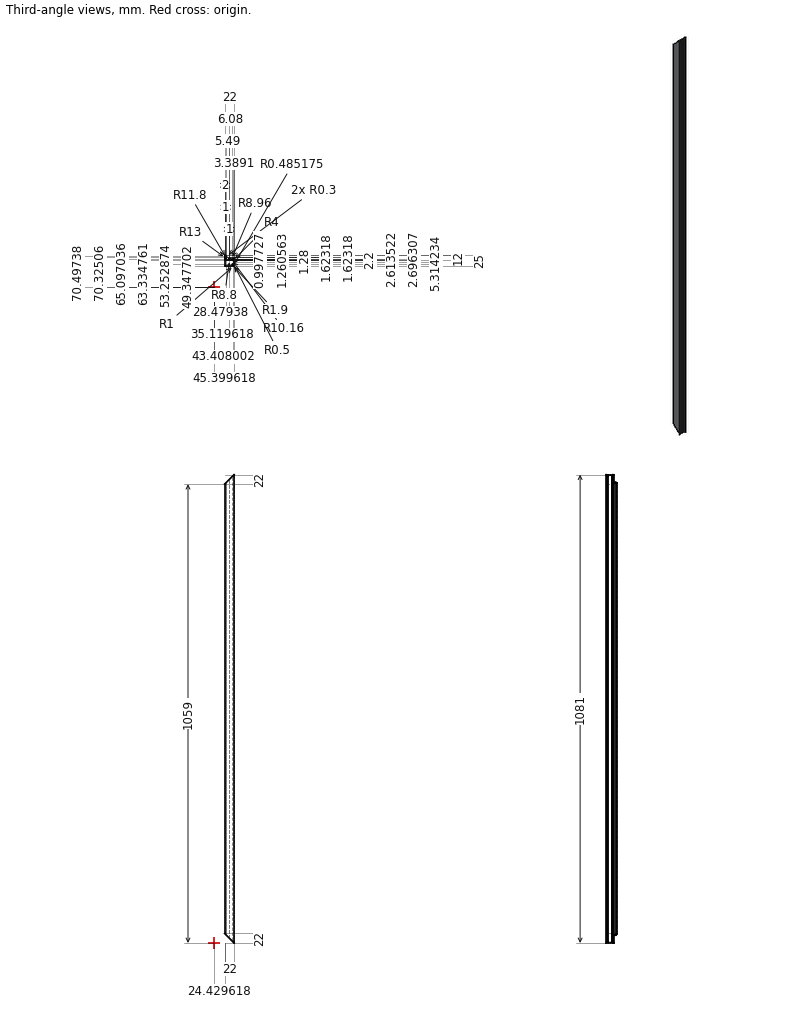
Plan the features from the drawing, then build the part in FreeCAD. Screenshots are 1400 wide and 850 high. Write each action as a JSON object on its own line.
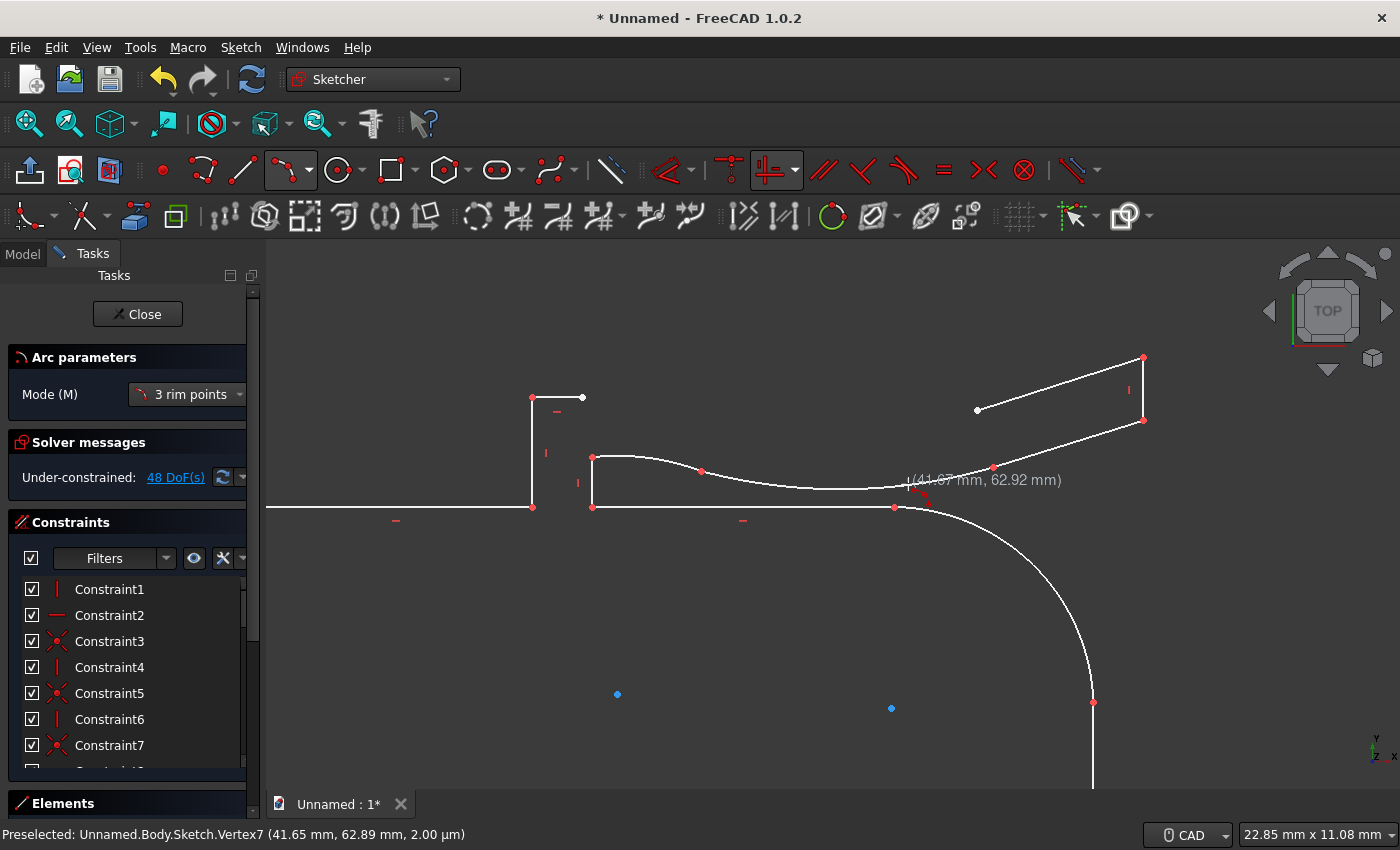
{"action": "left_click", "coordinate": [977, 411]}
{"action": "left_click", "coordinate": [719, 412]}
{"action": "left_click", "coordinate": [848, 429]}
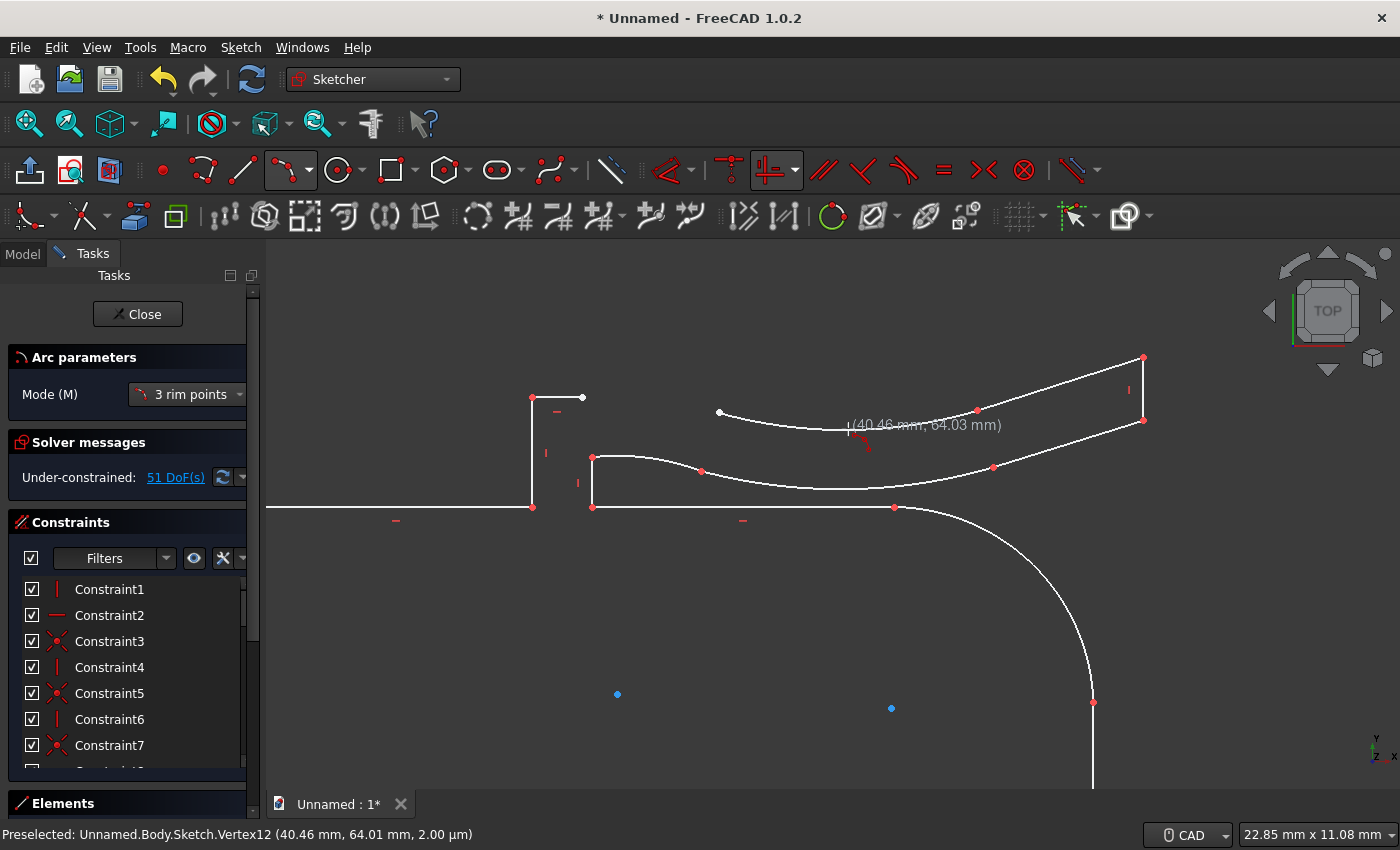
{"action": "left_click", "coordinate": [719, 413]}
{"action": "left_click", "coordinate": [582, 397]}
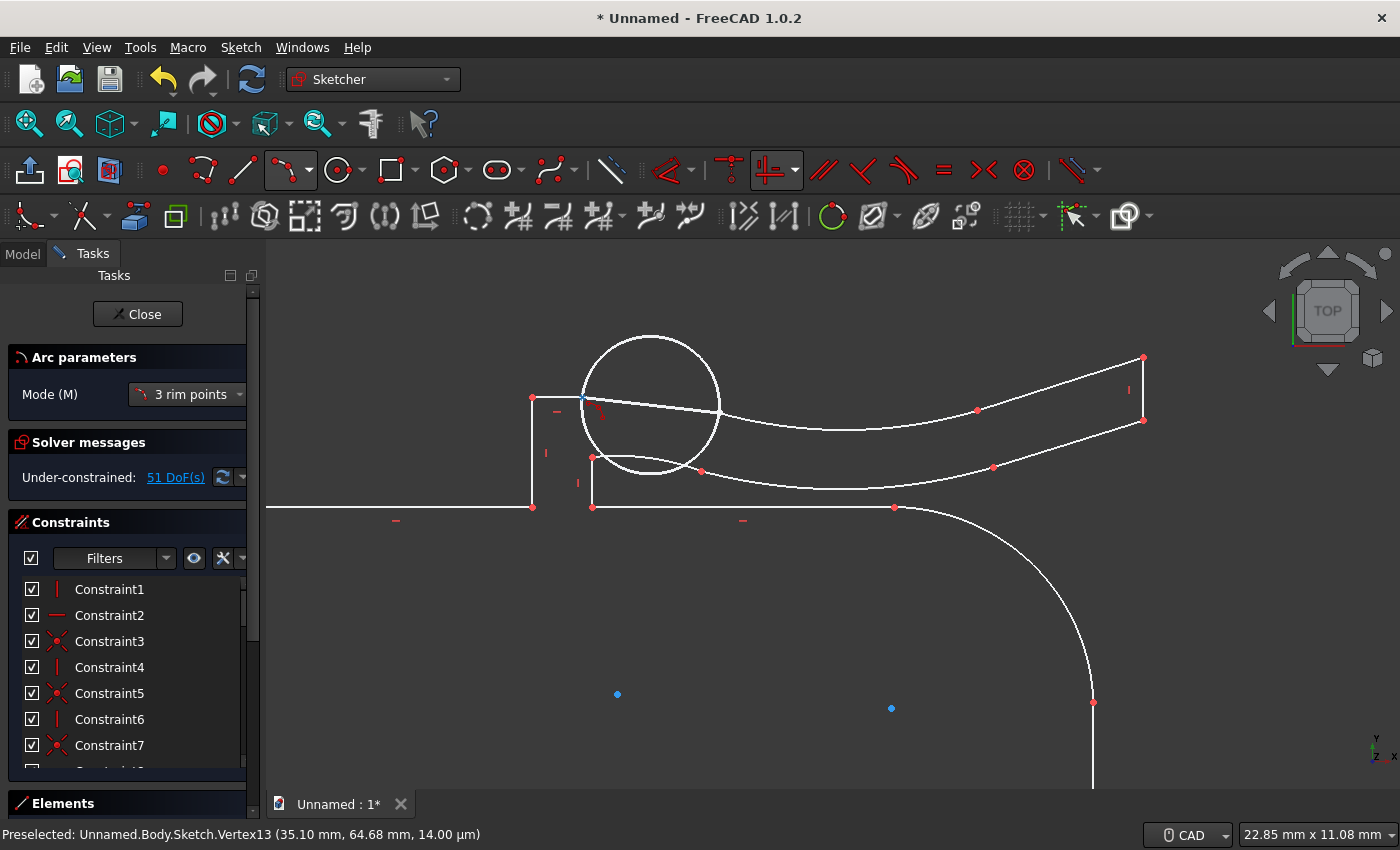
{"action": "scroll", "coordinate": [651, 398], "scroll_direction": "up", "scroll_amount": 7}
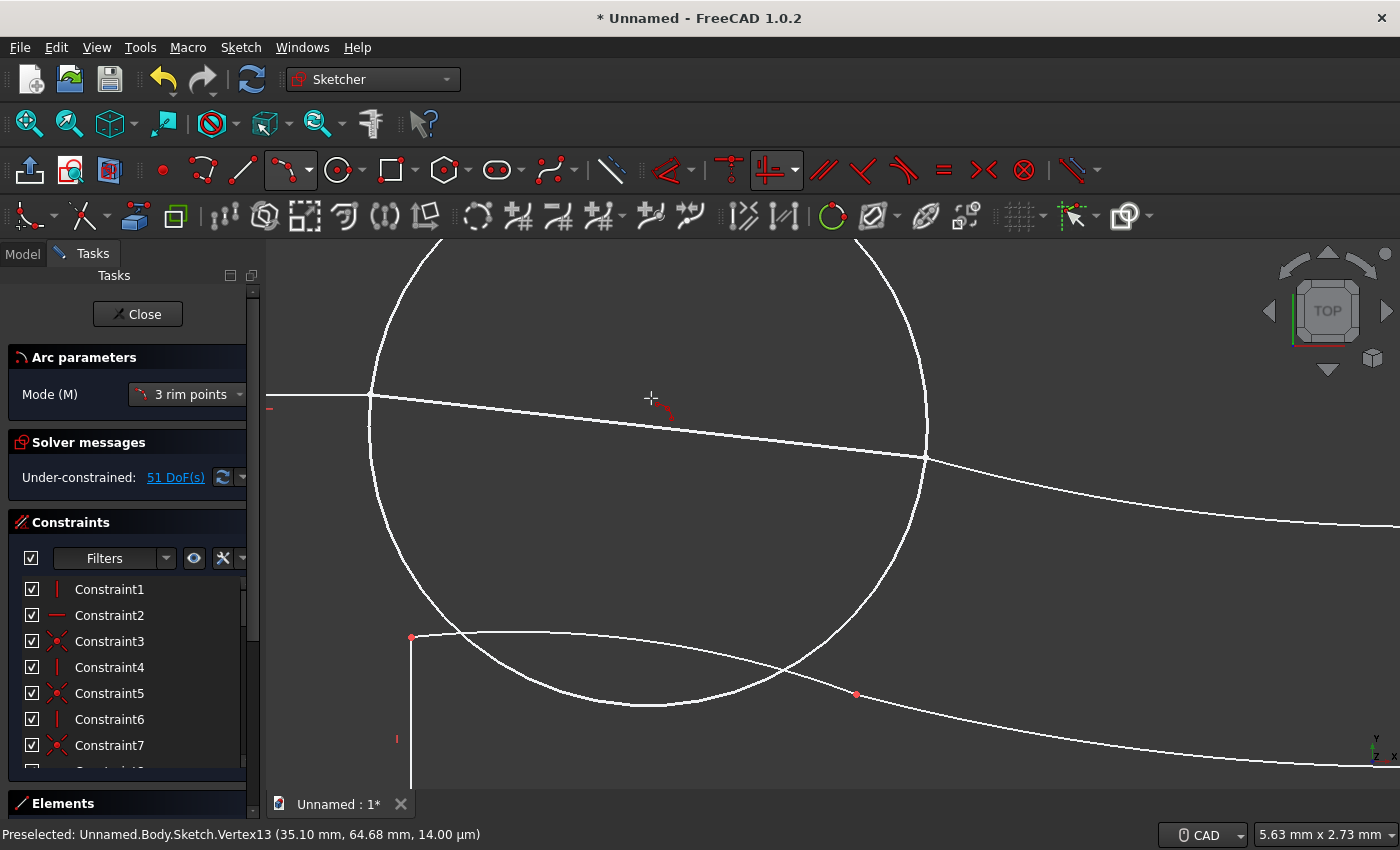
{"action": "left_click", "coordinate": [652, 397]}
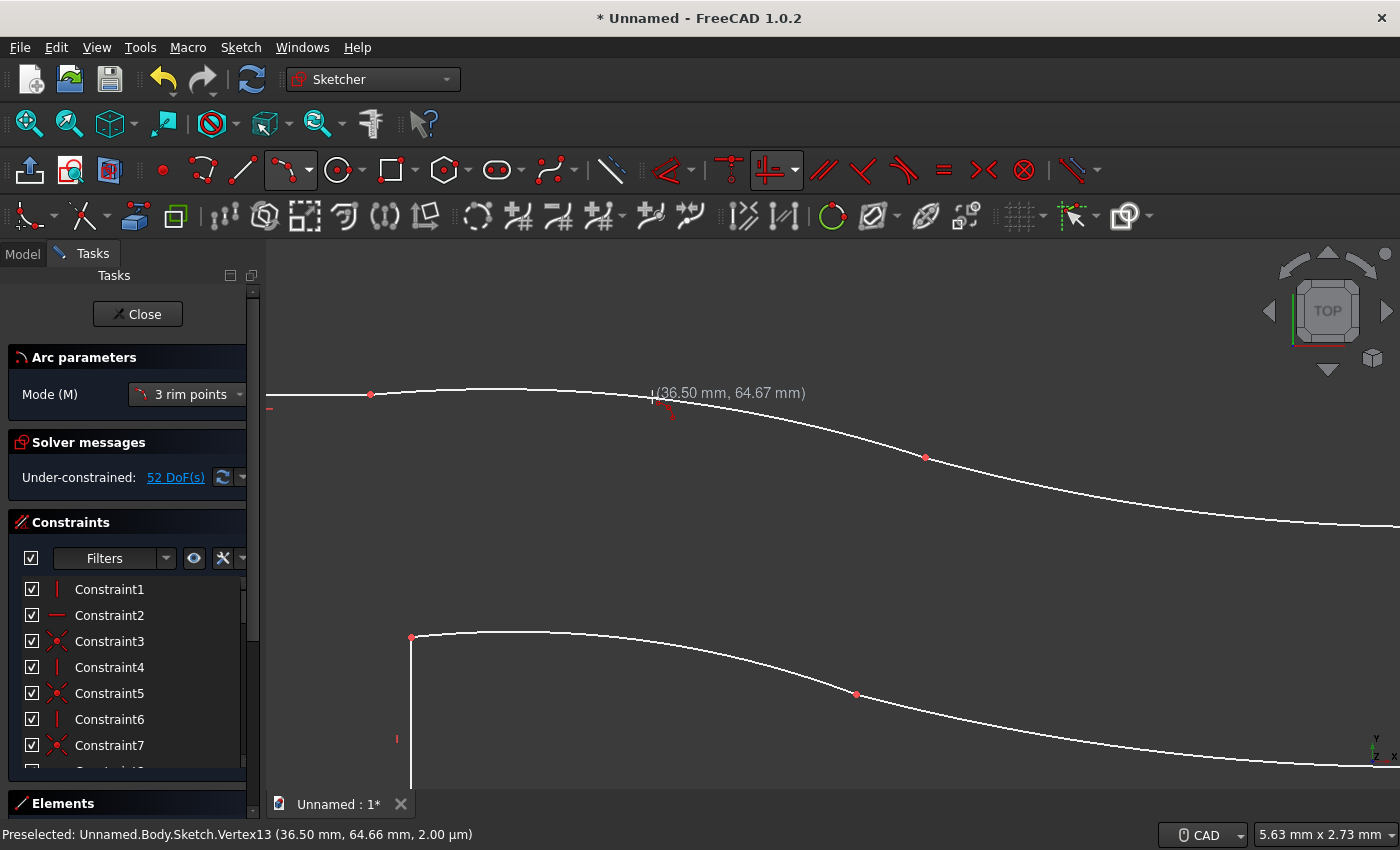
{"action": "scroll", "coordinate": [791, 459], "scroll_direction": "down", "scroll_amount": 13}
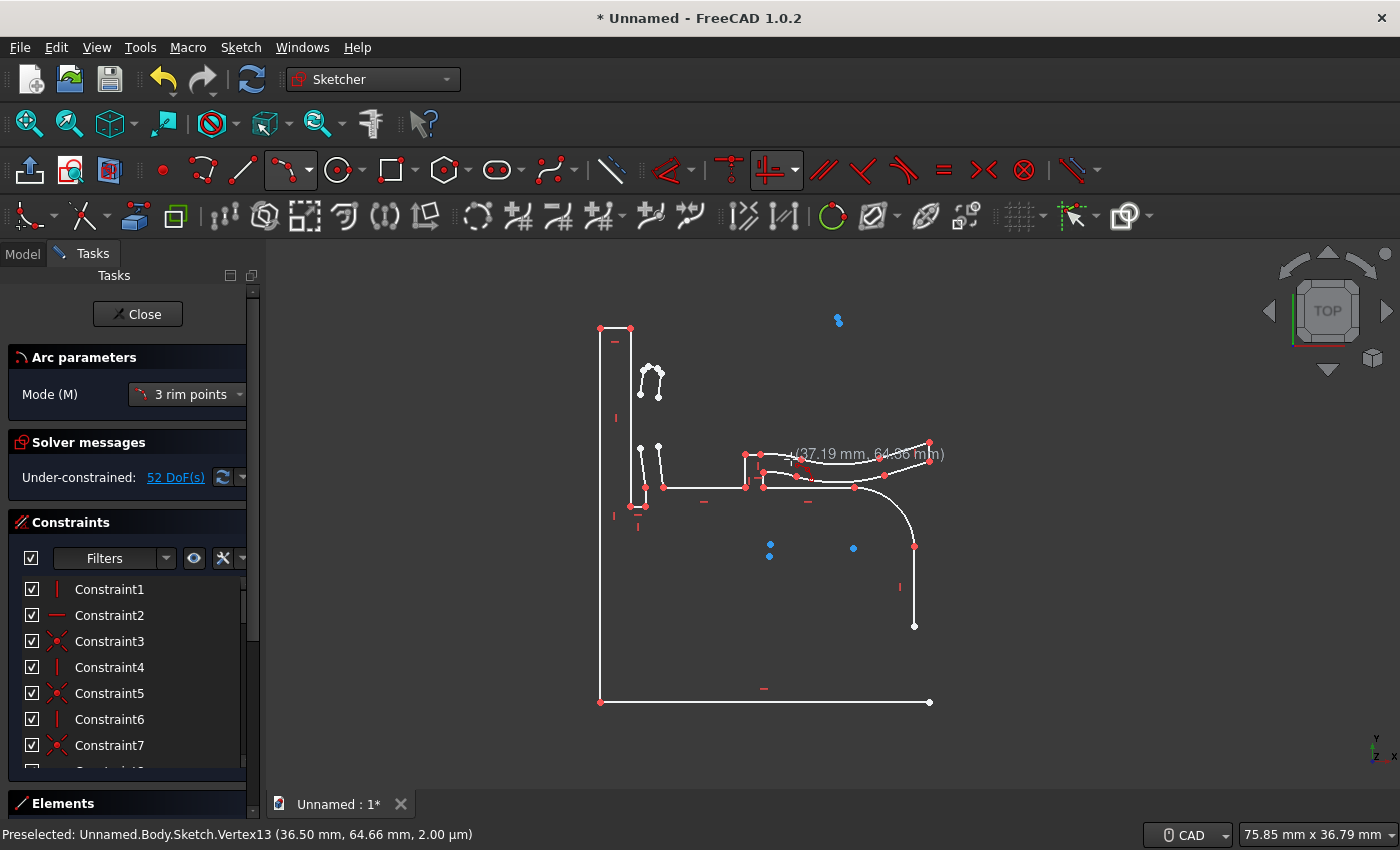
{"action": "left_click", "coordinate": [658, 447]}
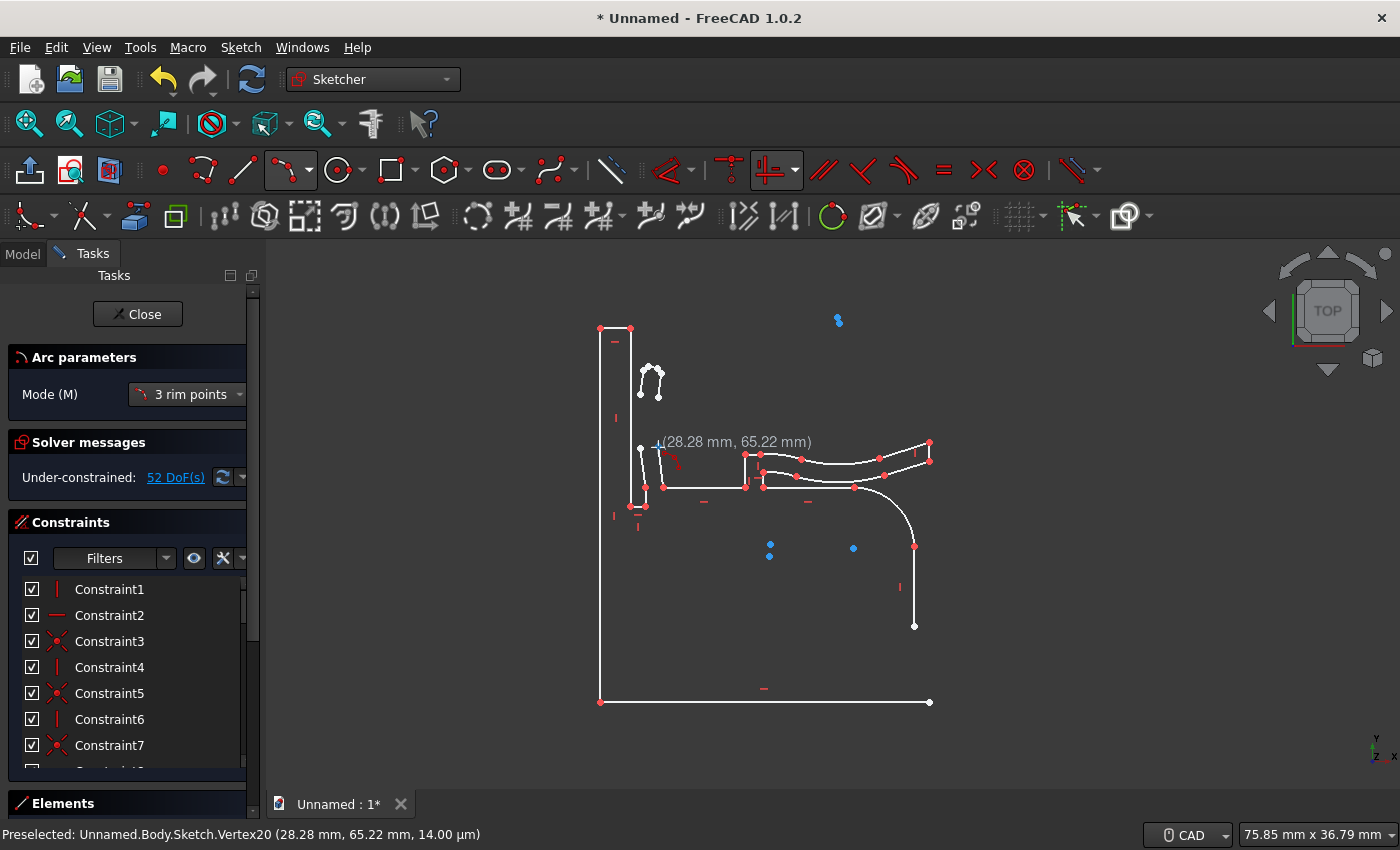
{"action": "scroll", "coordinate": [658, 397], "scroll_direction": "up", "scroll_amount": 2}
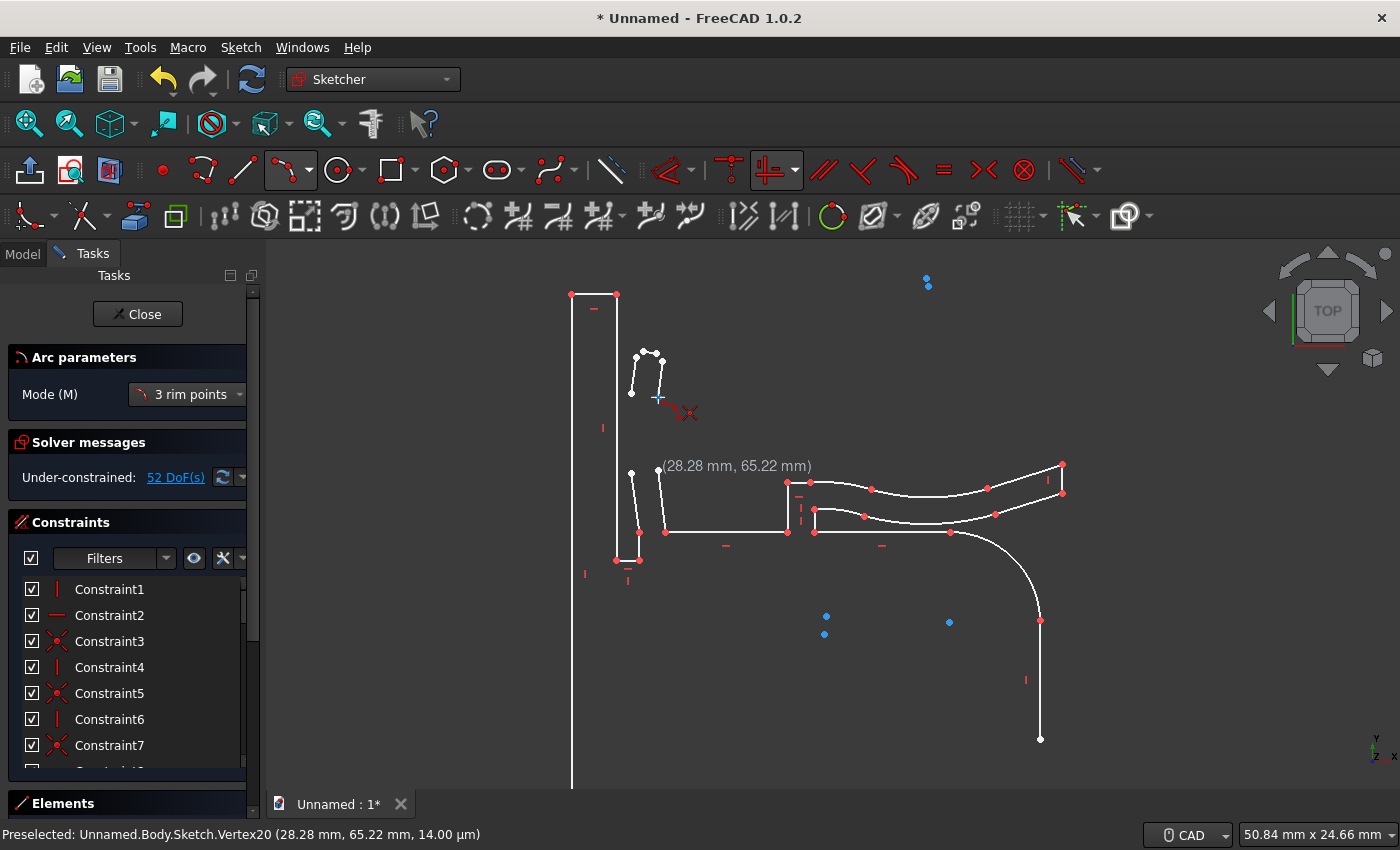
{"action": "left_click", "coordinate": [658, 398]}